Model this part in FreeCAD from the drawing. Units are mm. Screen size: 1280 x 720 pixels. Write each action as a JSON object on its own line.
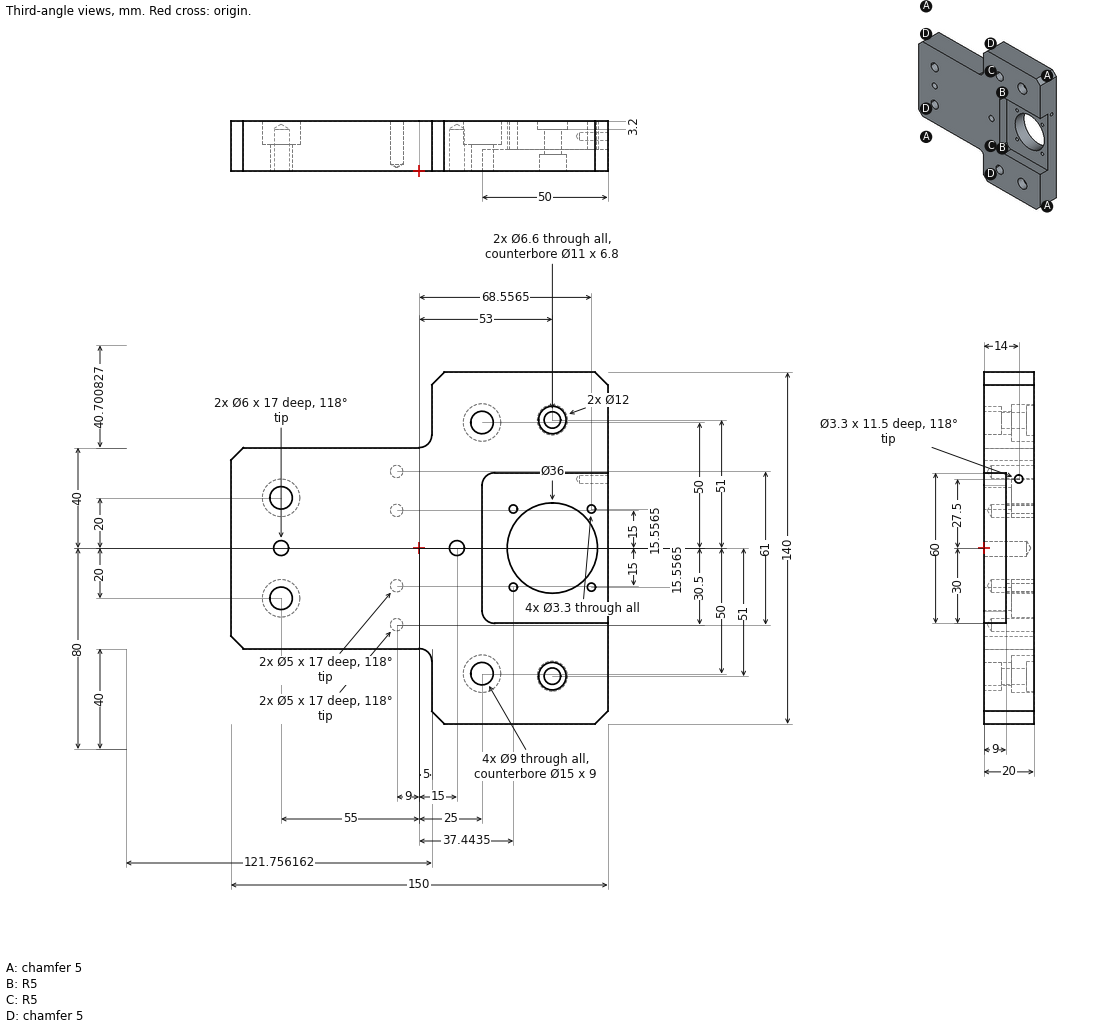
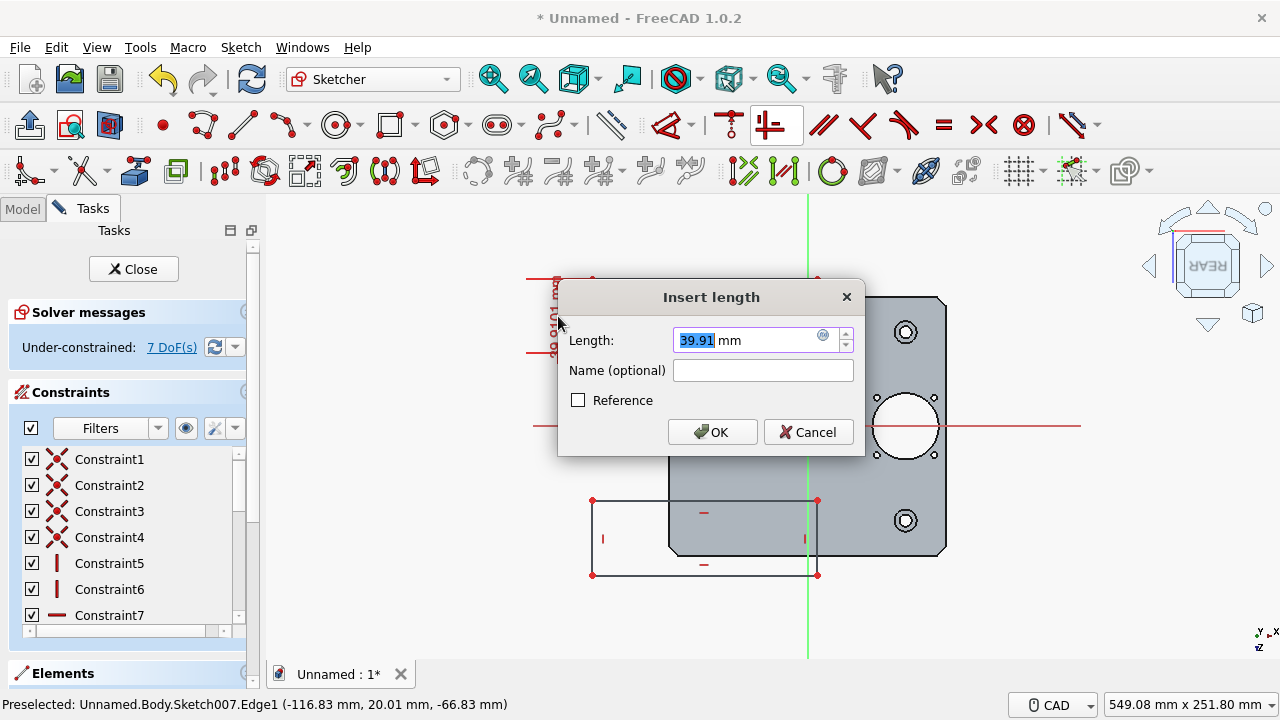
{"action": "type", "text": "40"}
{"action": "key", "text": "Return"}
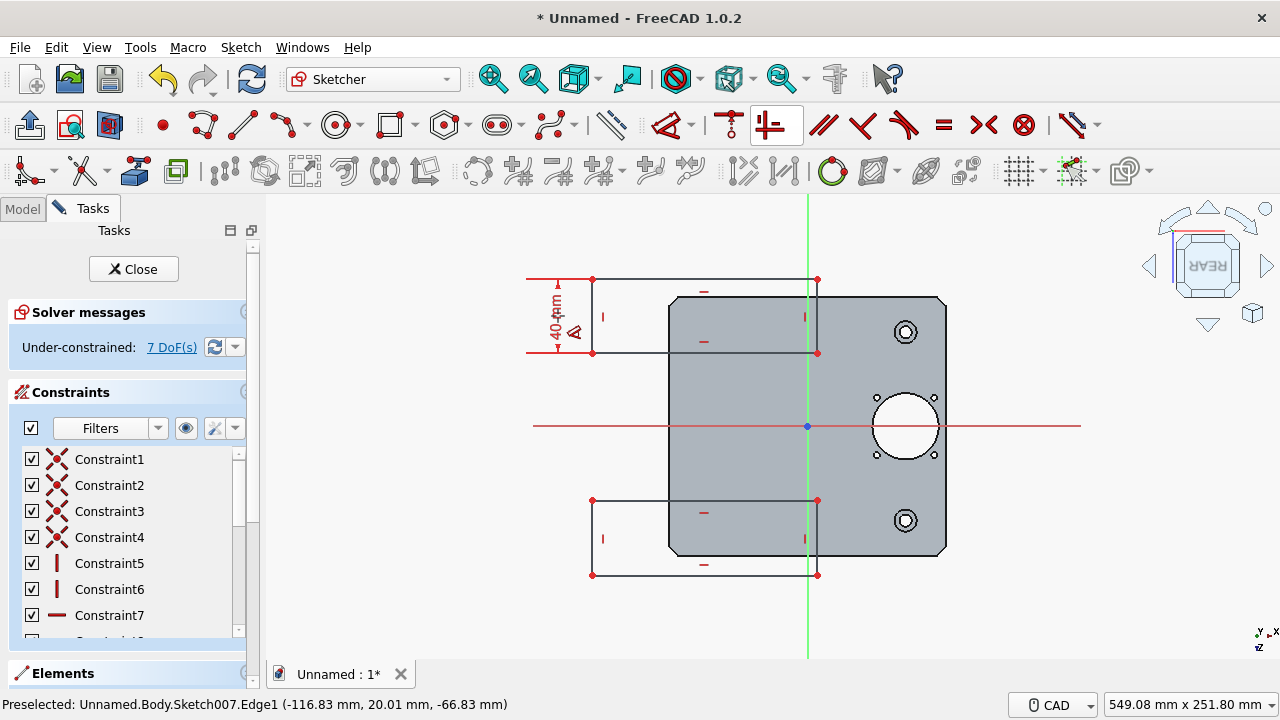
{"action": "scroll", "coordinate": [817, 353], "scroll_direction": "up", "scroll_amount": 8}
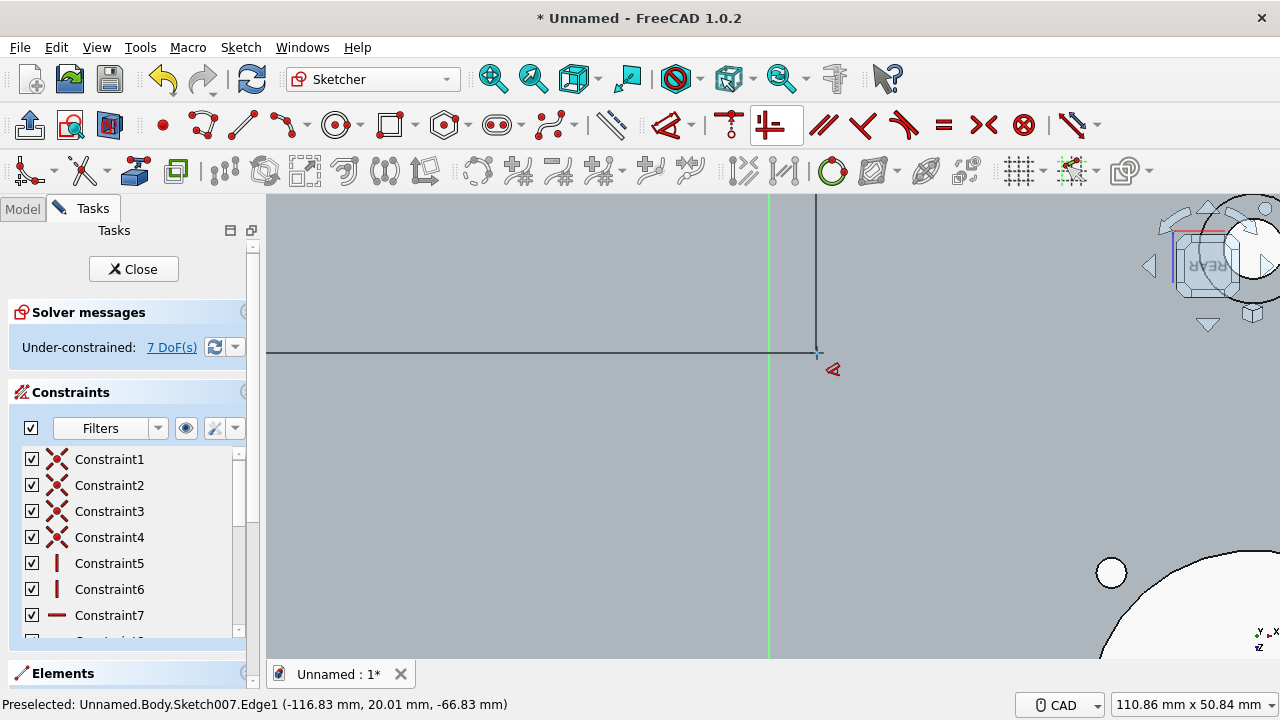
{"action": "left_click", "coordinate": [816, 353]}
{"action": "left_click", "coordinate": [793, 319]}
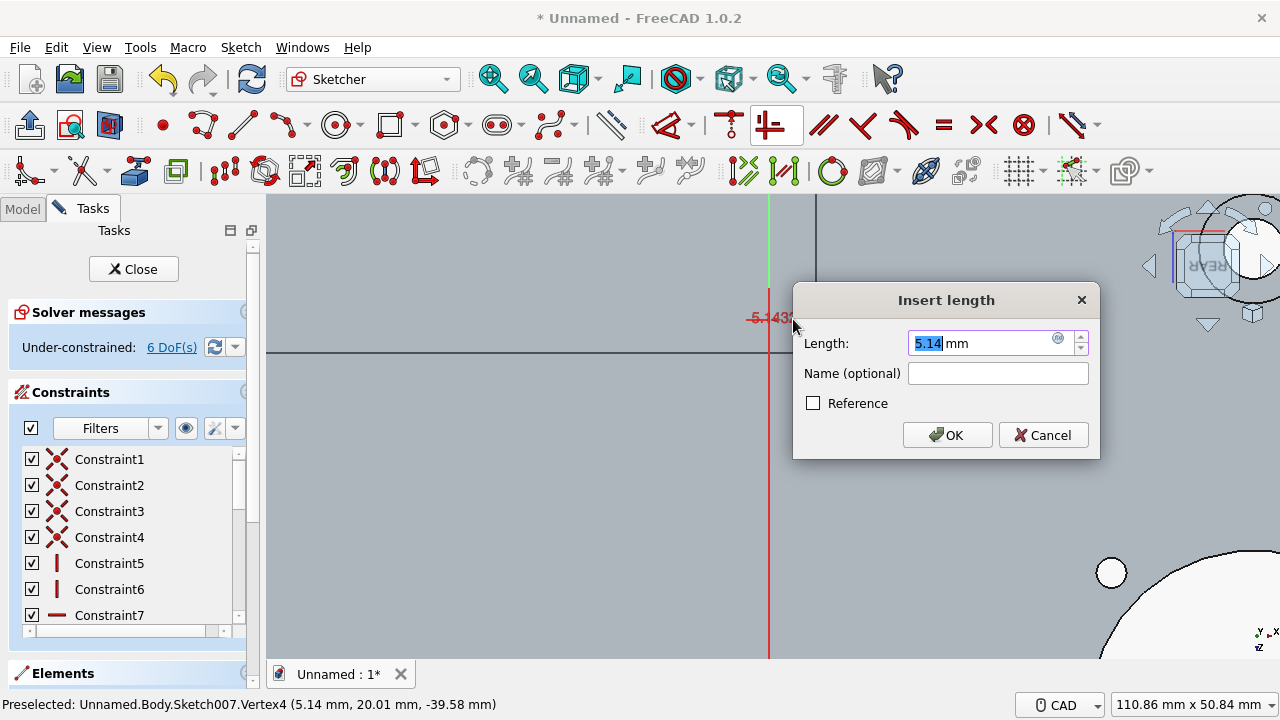
{"action": "type", "text": "5"}
{"action": "key", "text": "Return"}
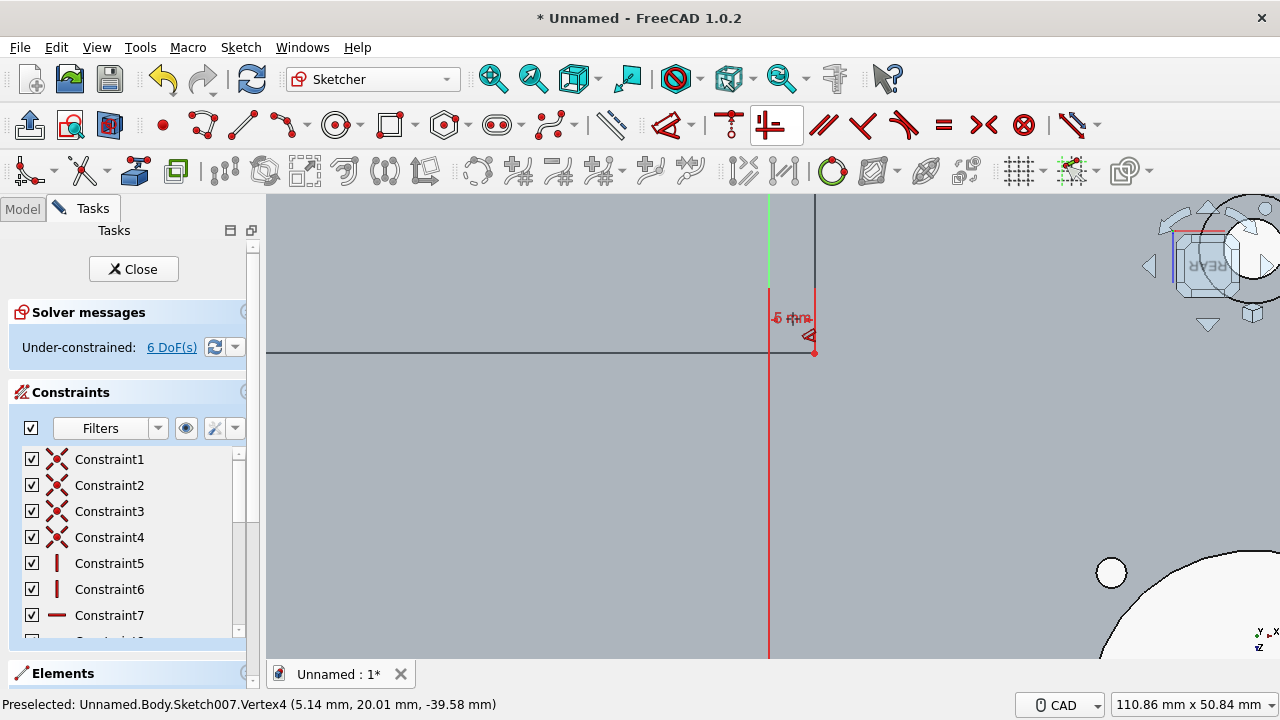
{"action": "scroll", "coordinate": [817, 353], "scroll_direction": "down", "scroll_amount": 8}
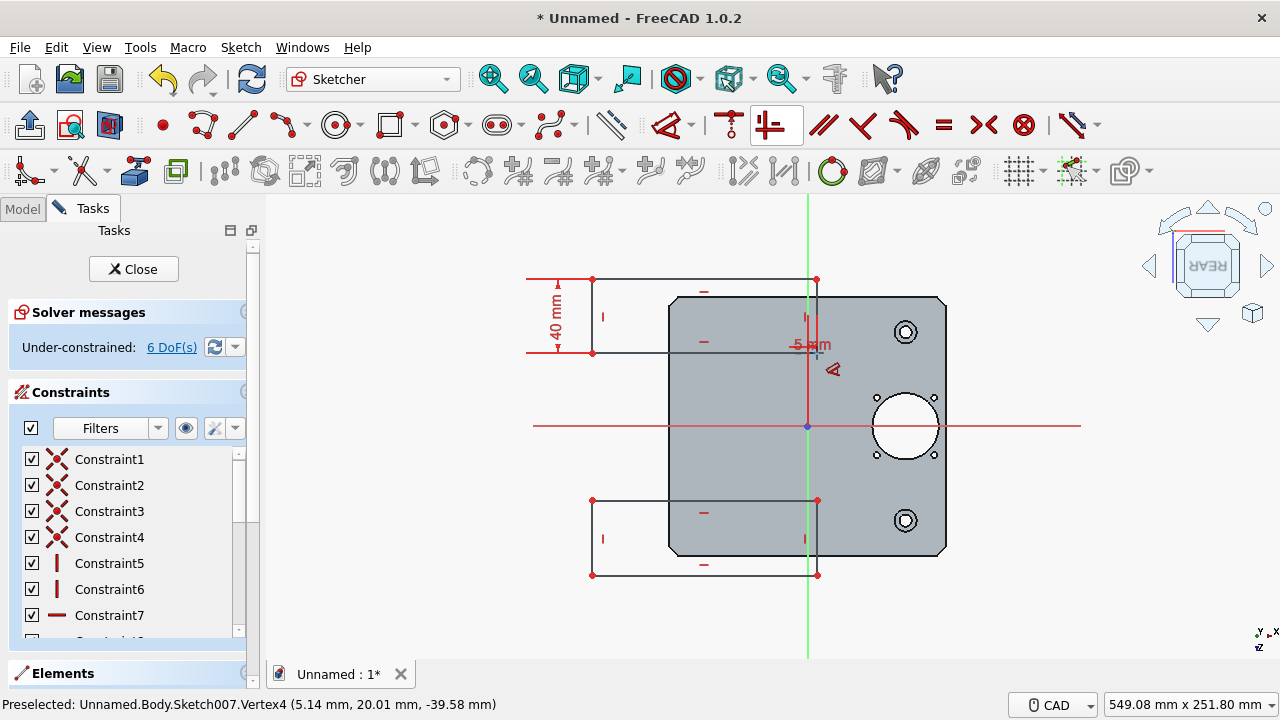
{"action": "scroll", "coordinate": [817, 576], "scroll_direction": "up", "scroll_amount": 8}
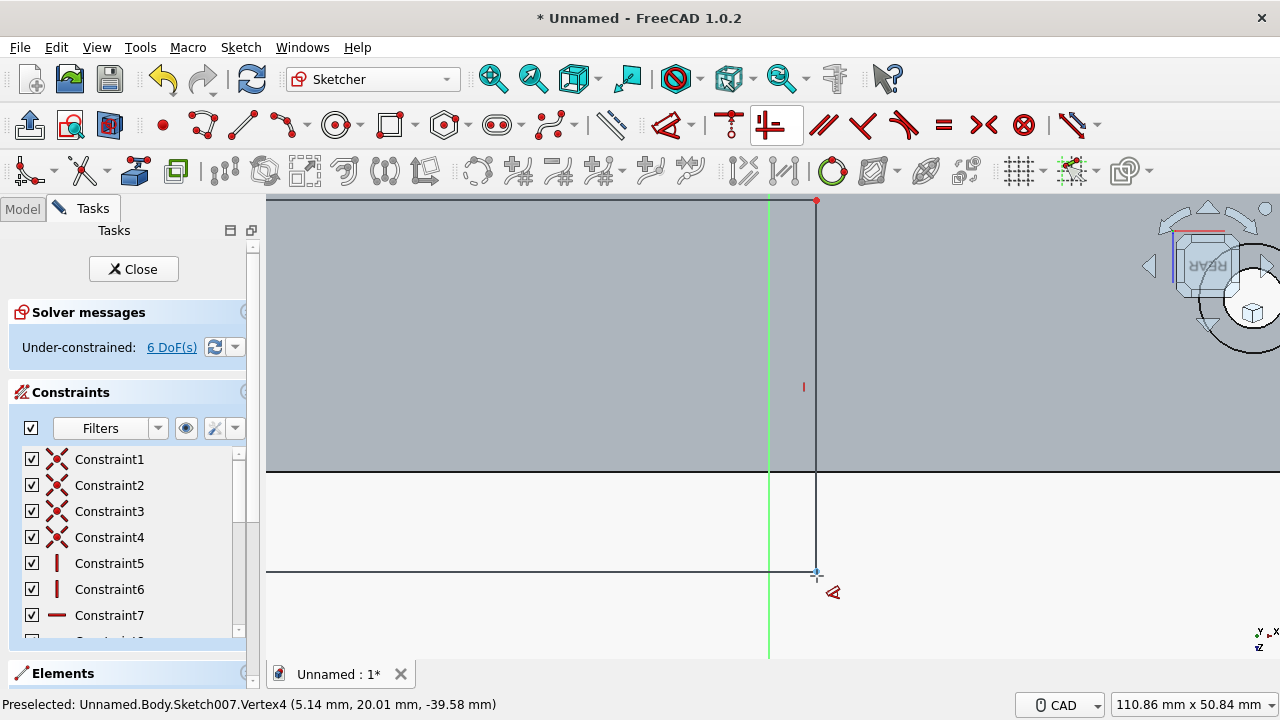
{"action": "left_click", "coordinate": [816, 572]}
{"action": "left_click", "coordinate": [793, 606]}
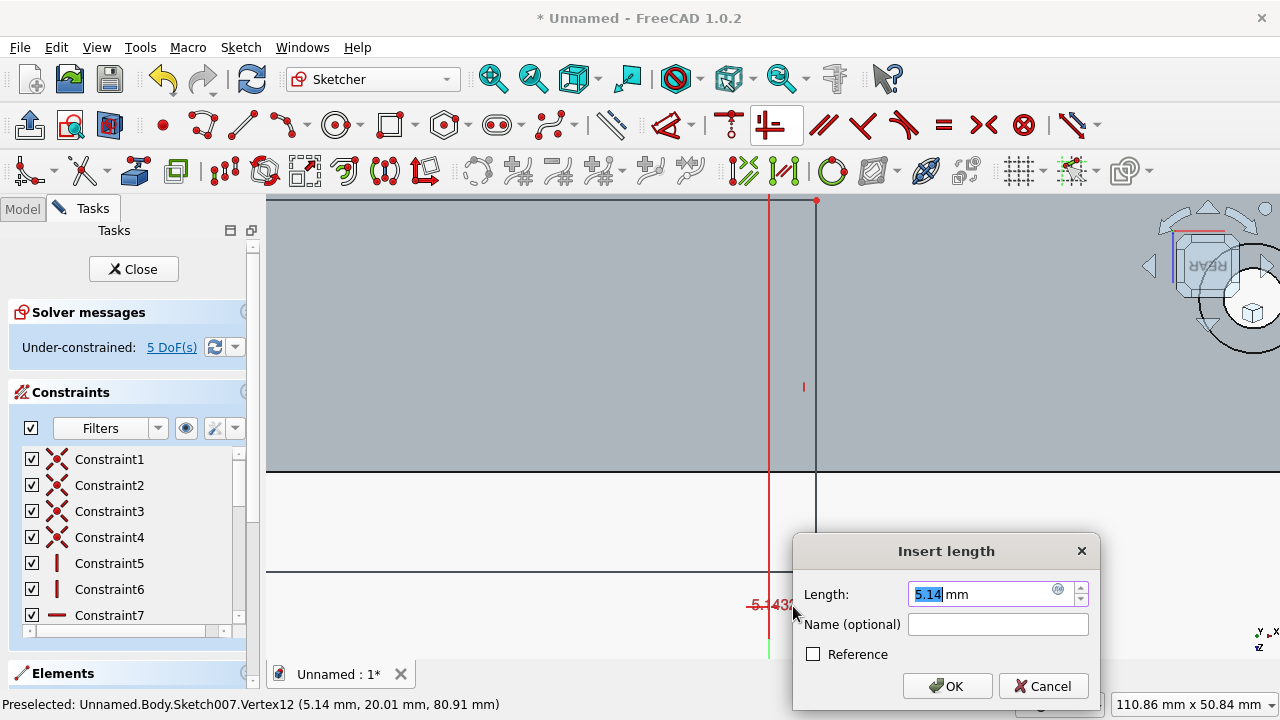
{"action": "type", "text": "5"}
{"action": "key", "text": "Return"}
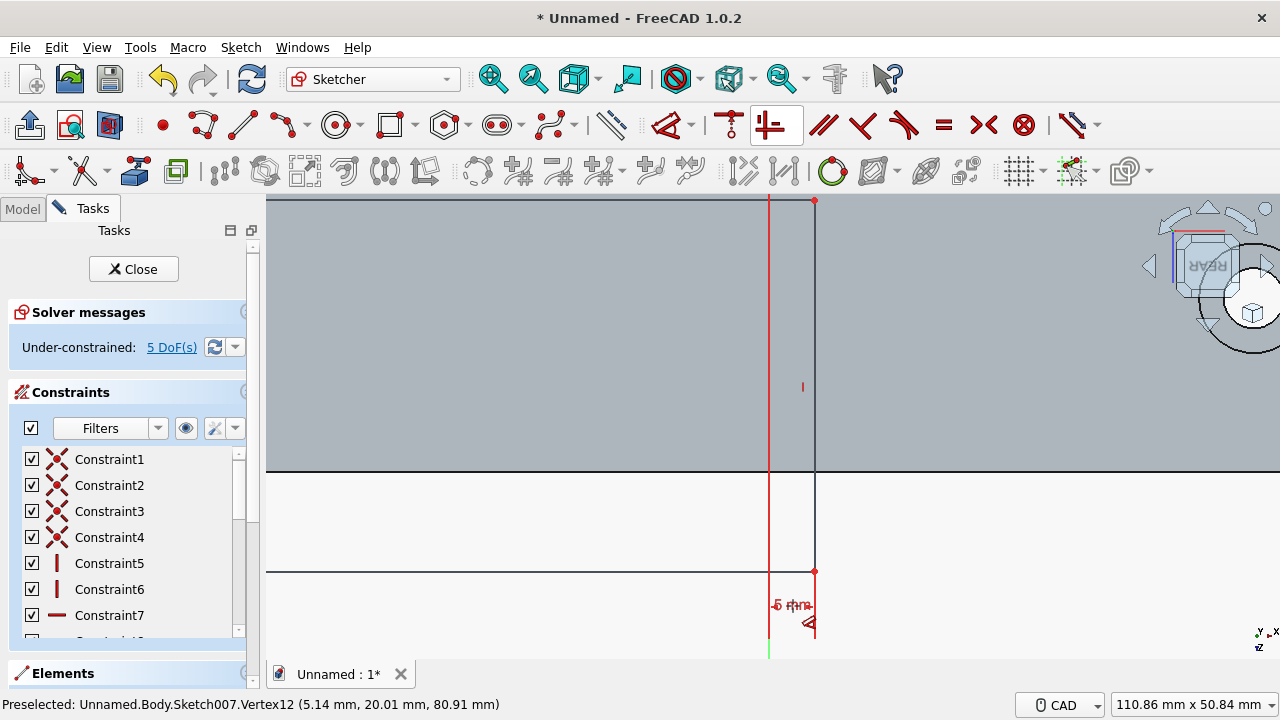
{"action": "scroll", "coordinate": [817, 576], "scroll_direction": "down", "scroll_amount": 8}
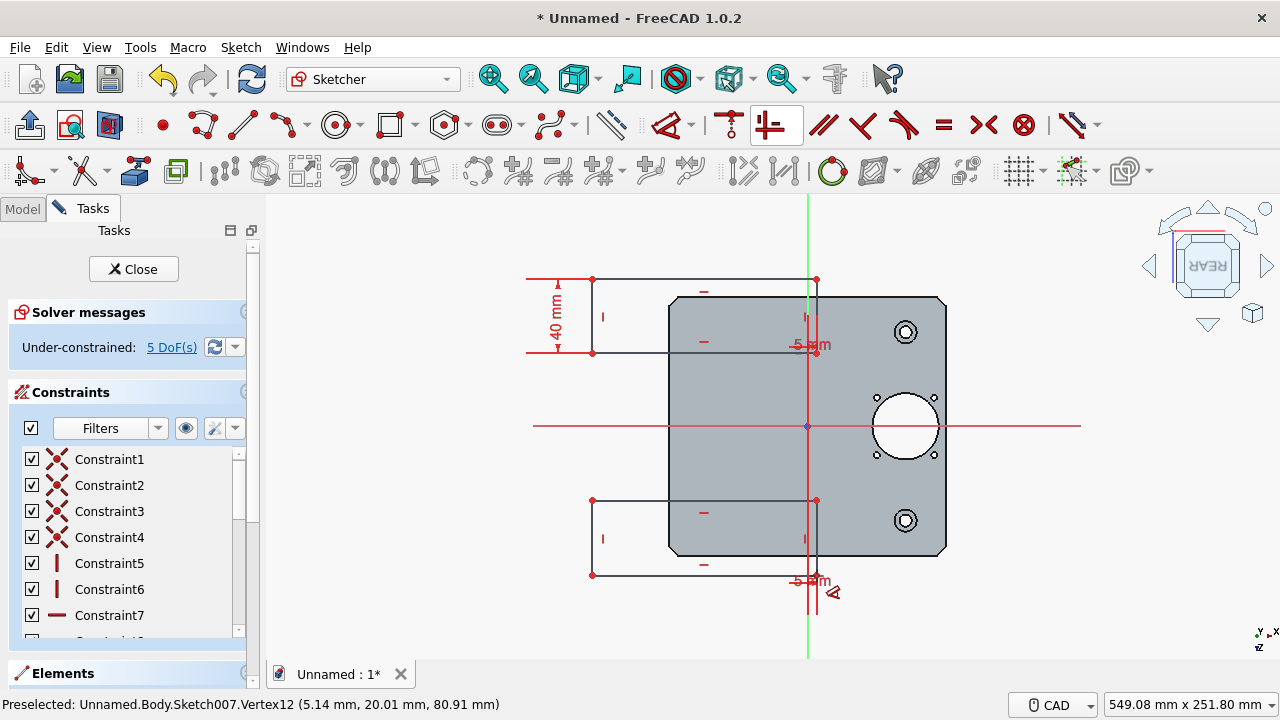
{"action": "left_click", "coordinate": [592, 279]}
{"action": "left_click", "coordinate": [558, 353]}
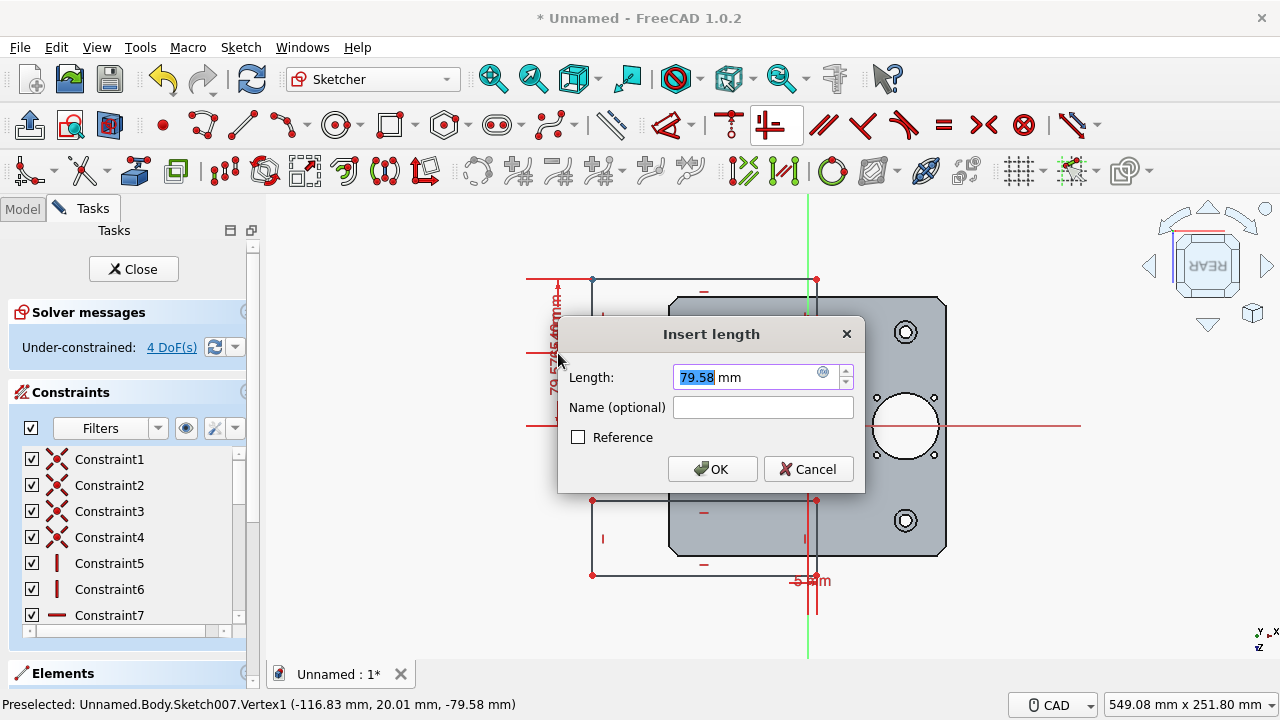
{"action": "type", "text": "80"}
{"action": "key", "text": "Return"}